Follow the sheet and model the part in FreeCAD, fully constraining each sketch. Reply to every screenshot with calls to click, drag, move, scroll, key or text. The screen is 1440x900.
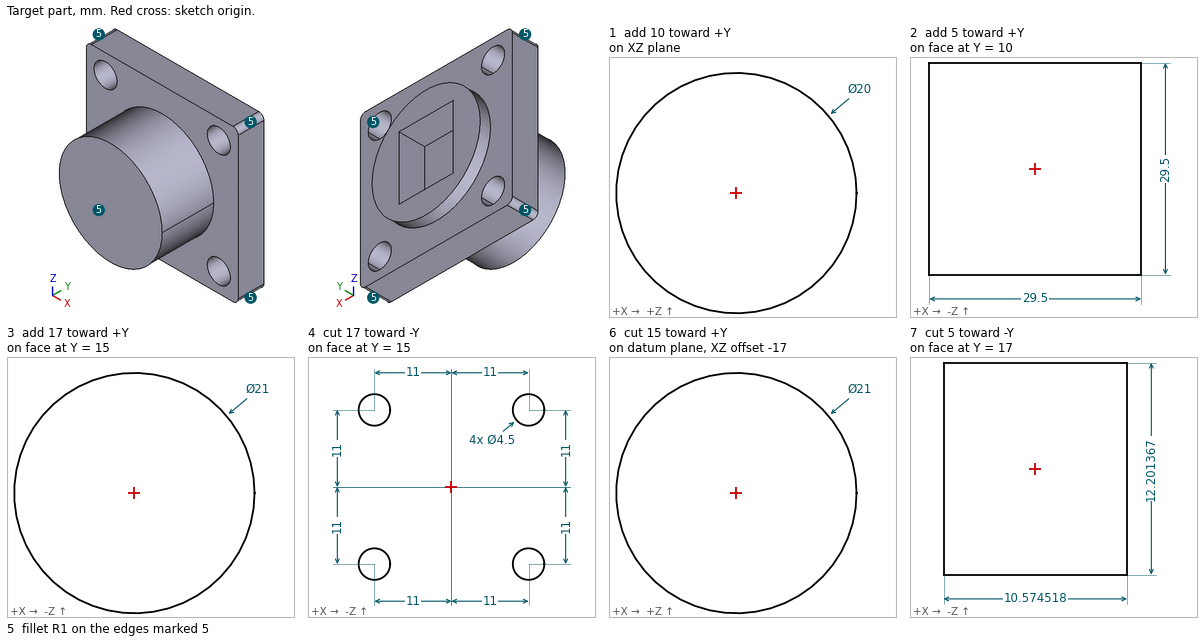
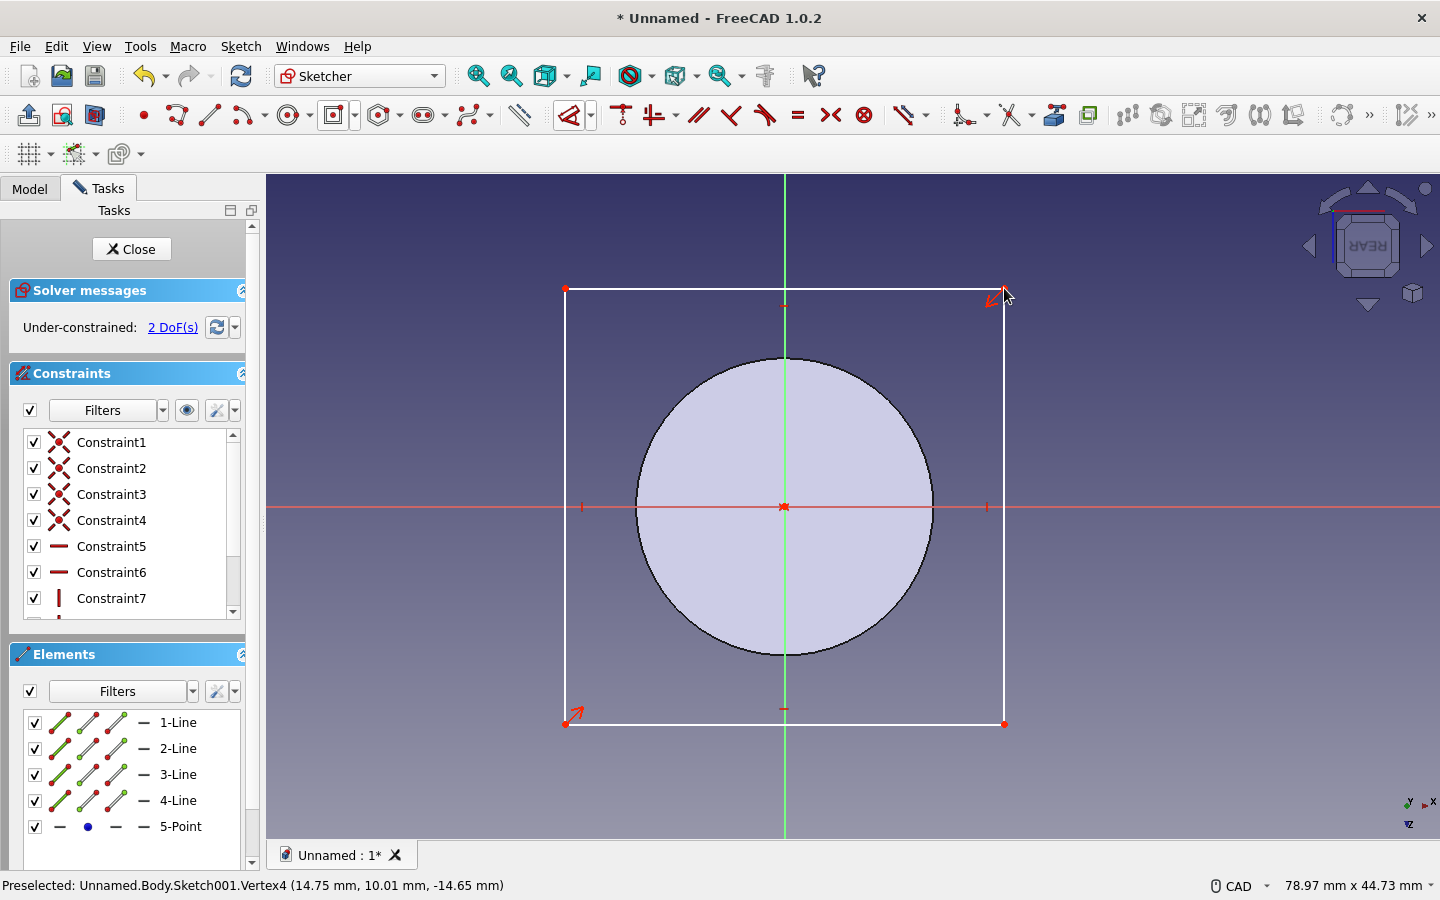
click(697, 725)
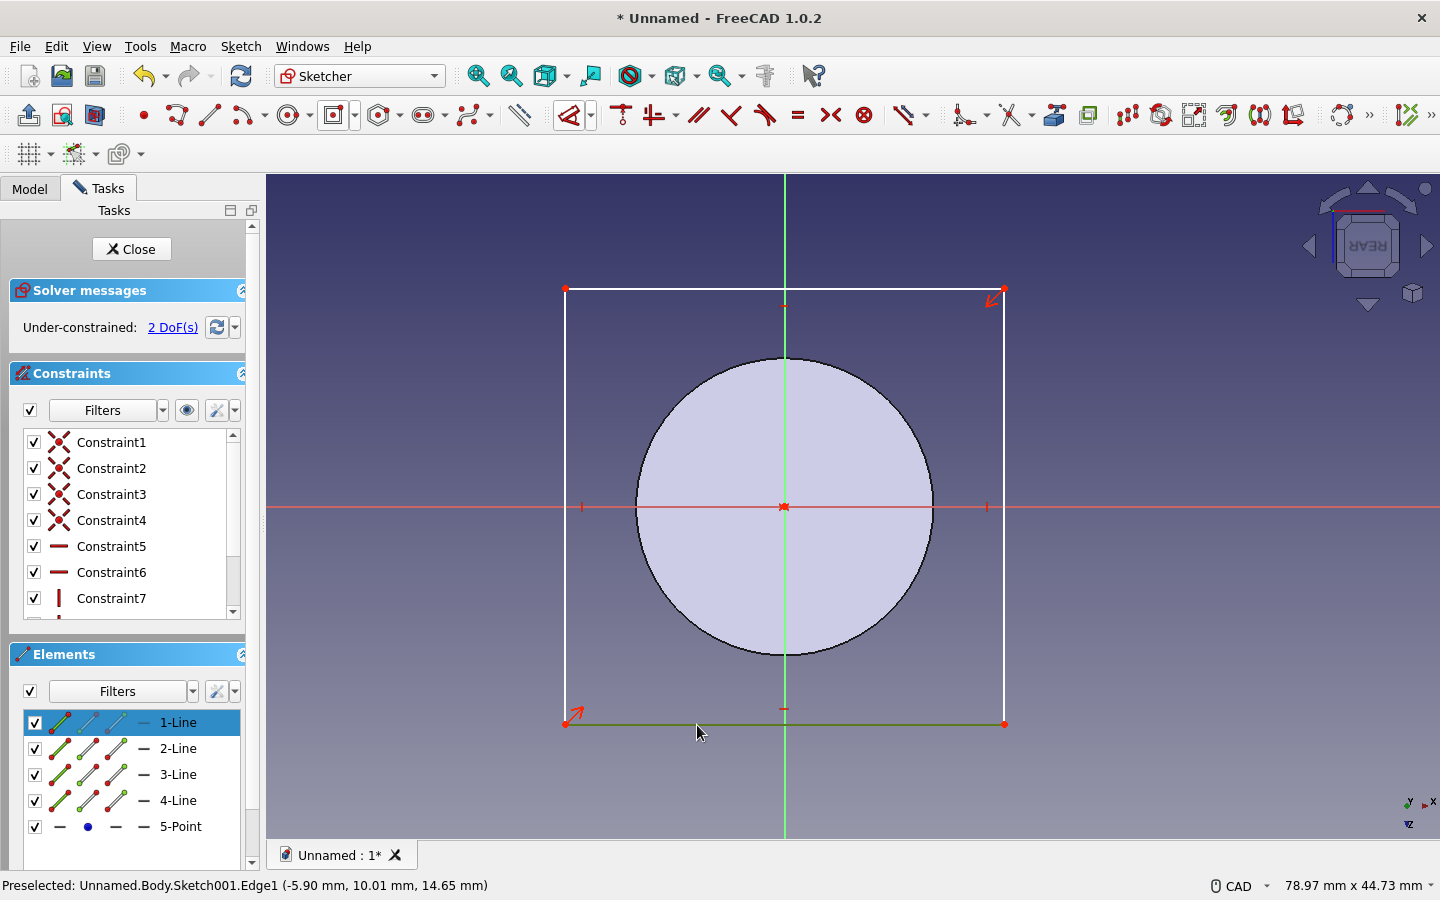
click(590, 116)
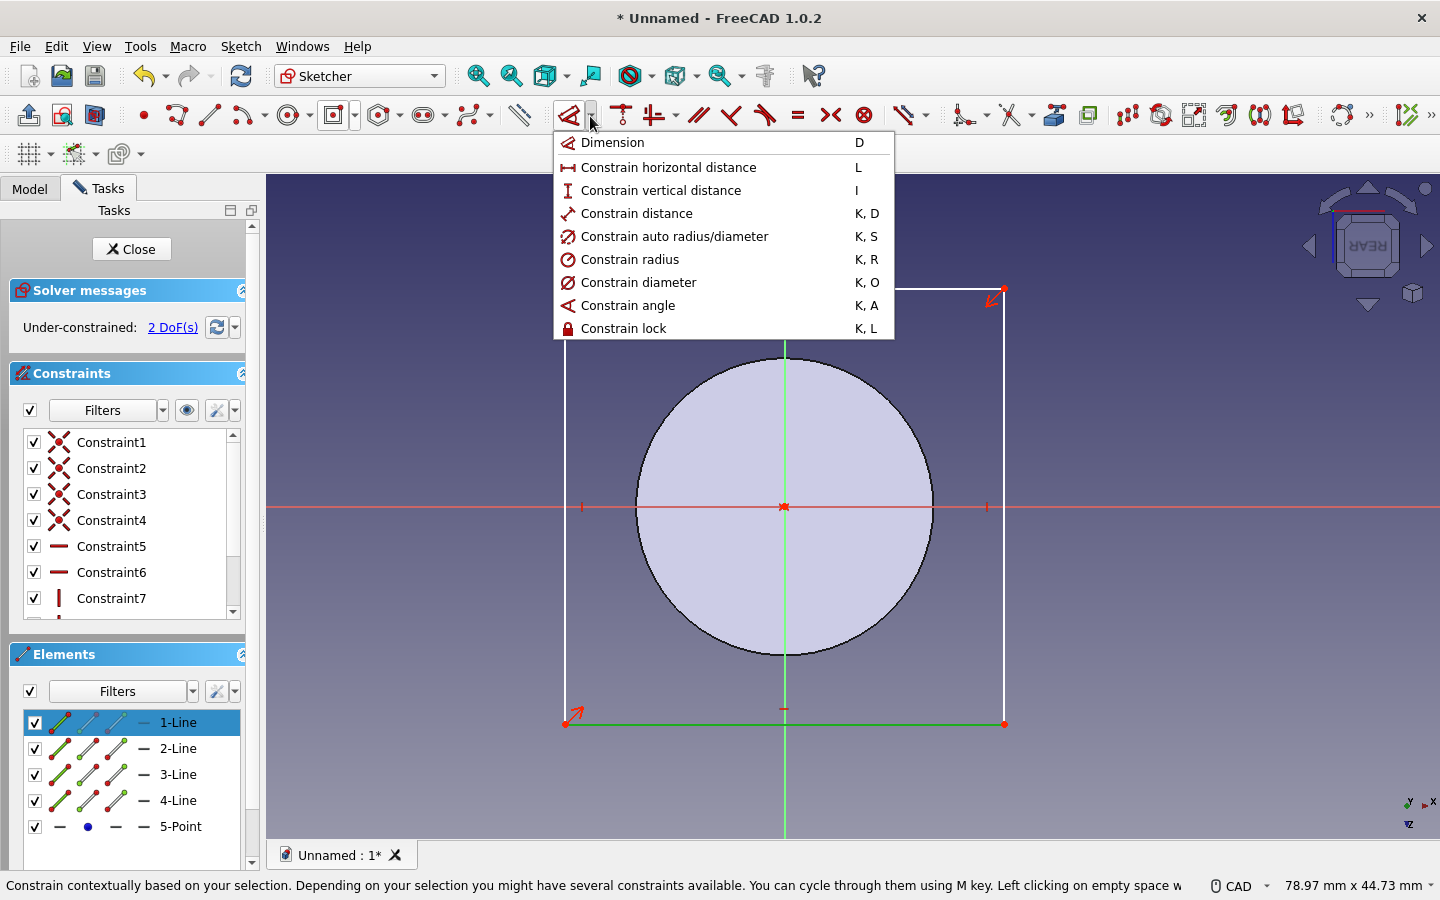
click(724, 168)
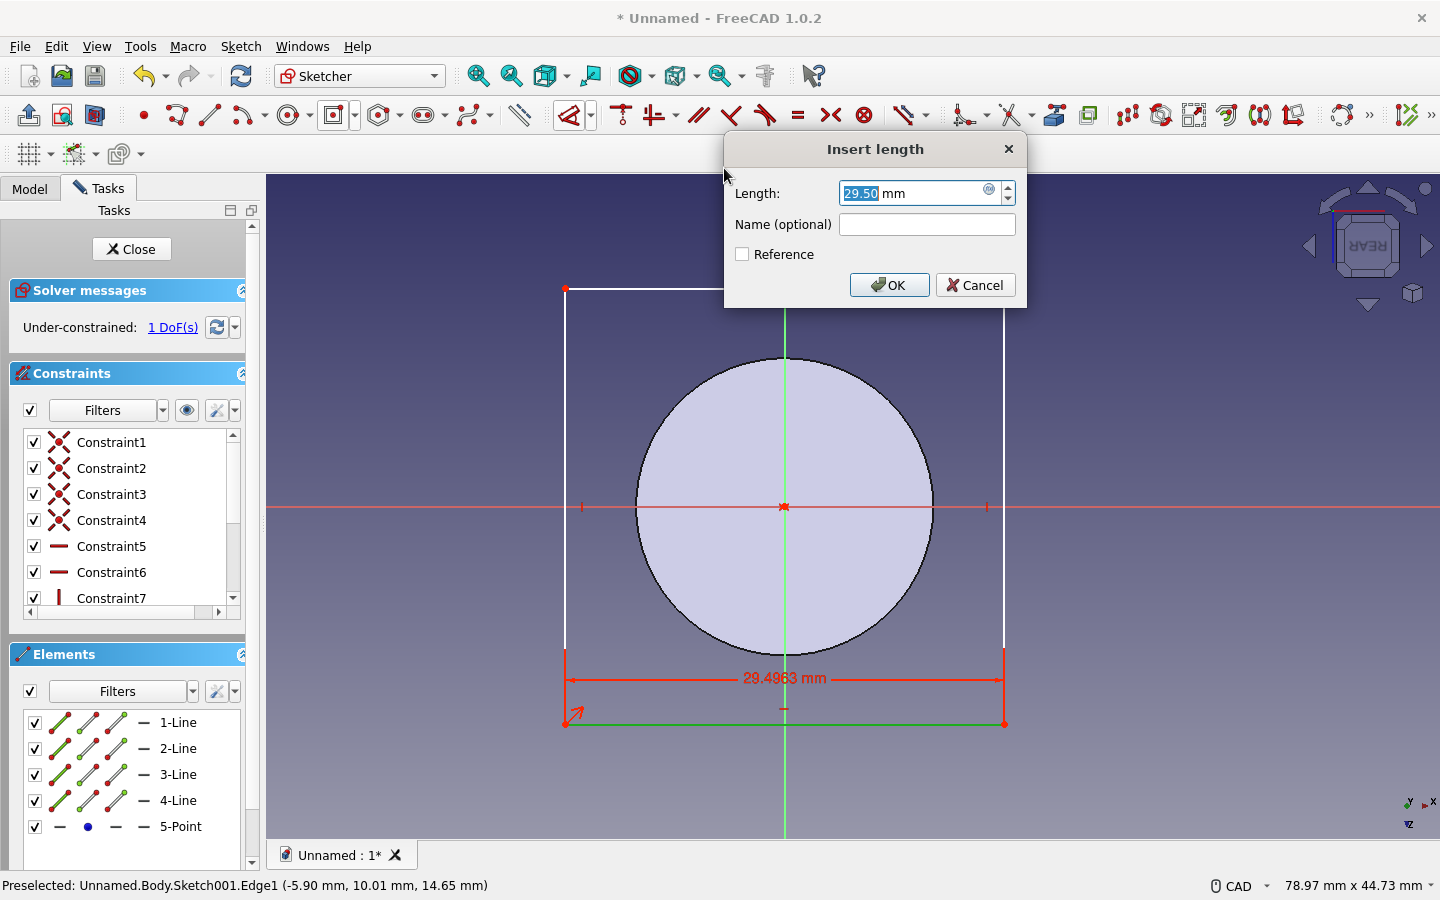
text(29.5)
key(Return)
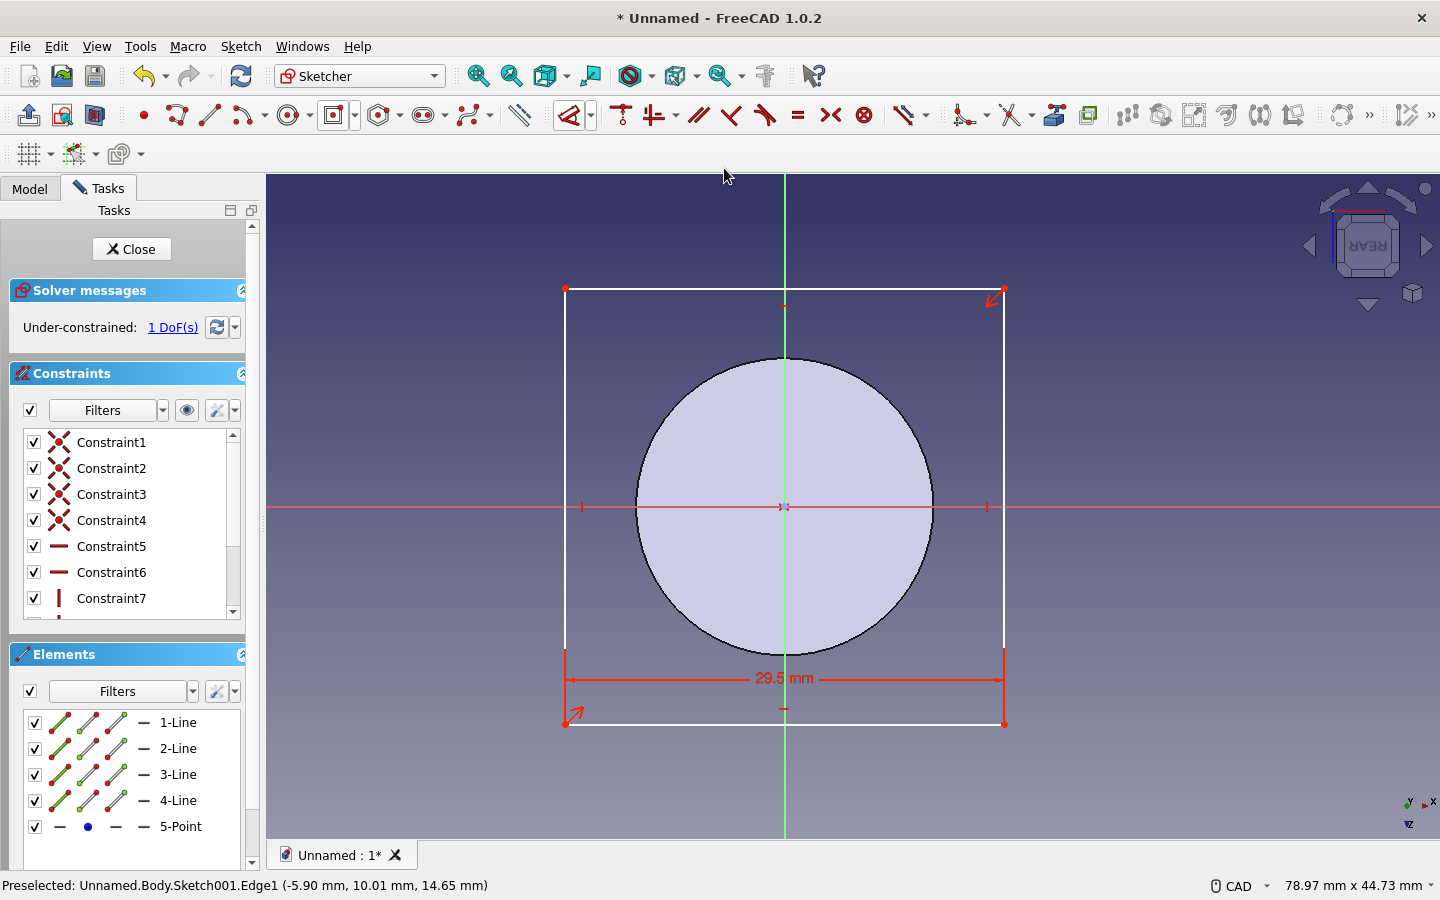
click(1004, 594)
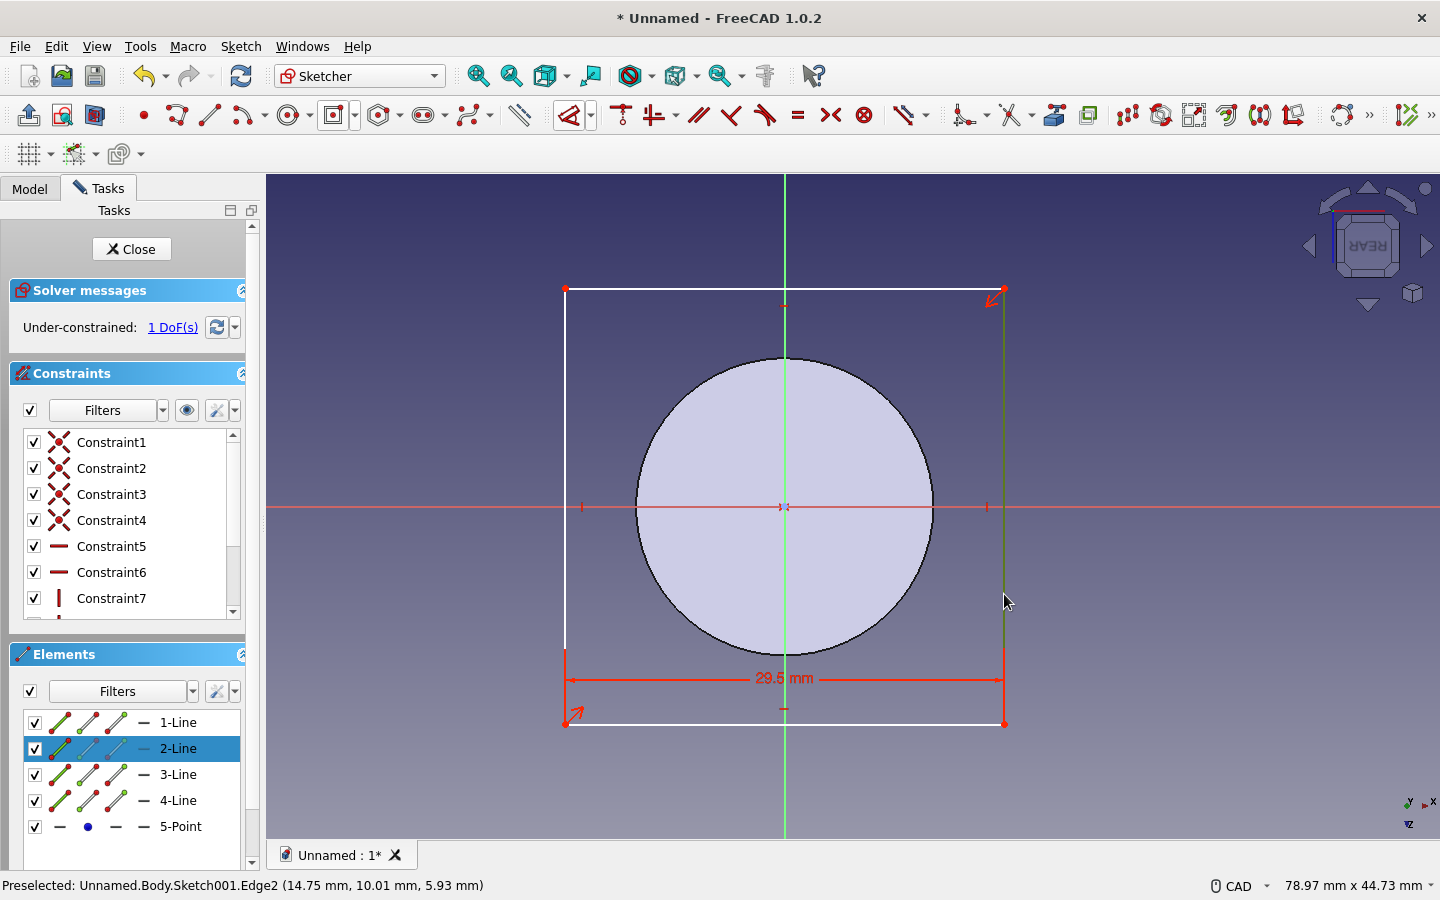
key(i)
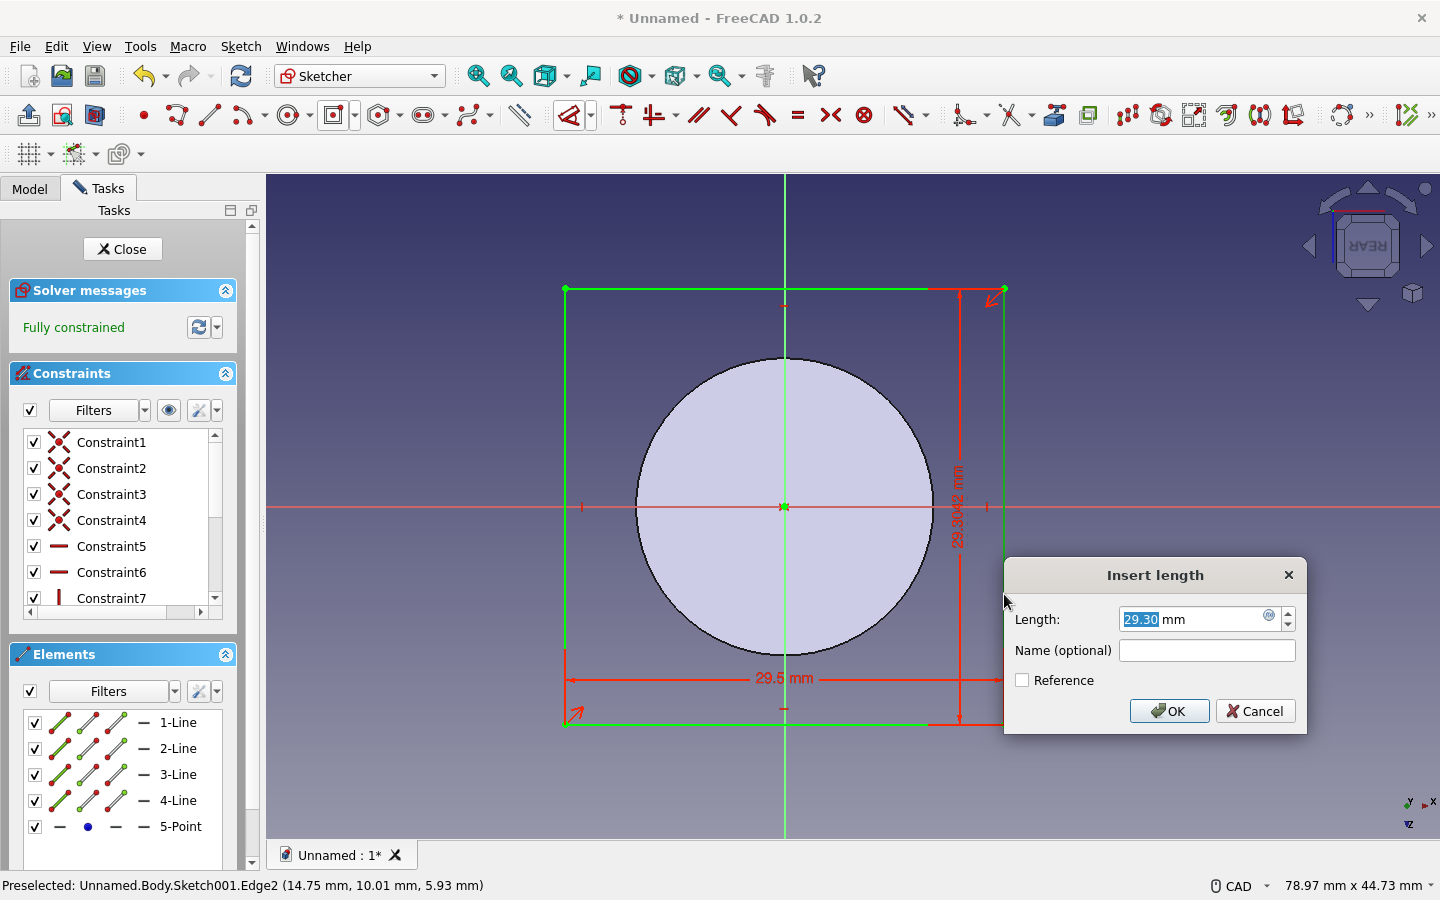
text(29.5)
key(Return)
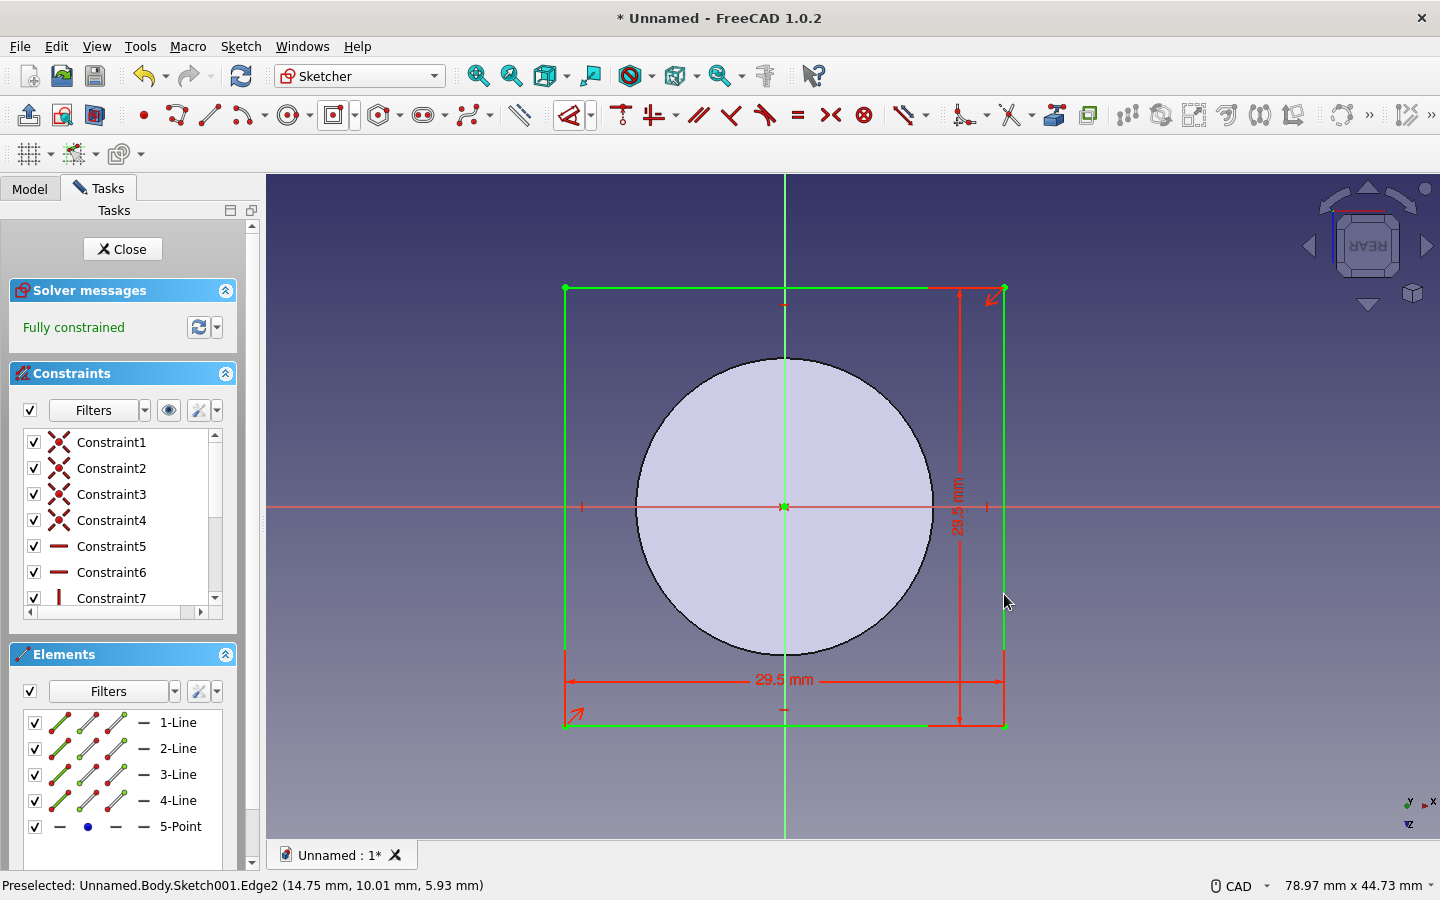
click(123, 249)